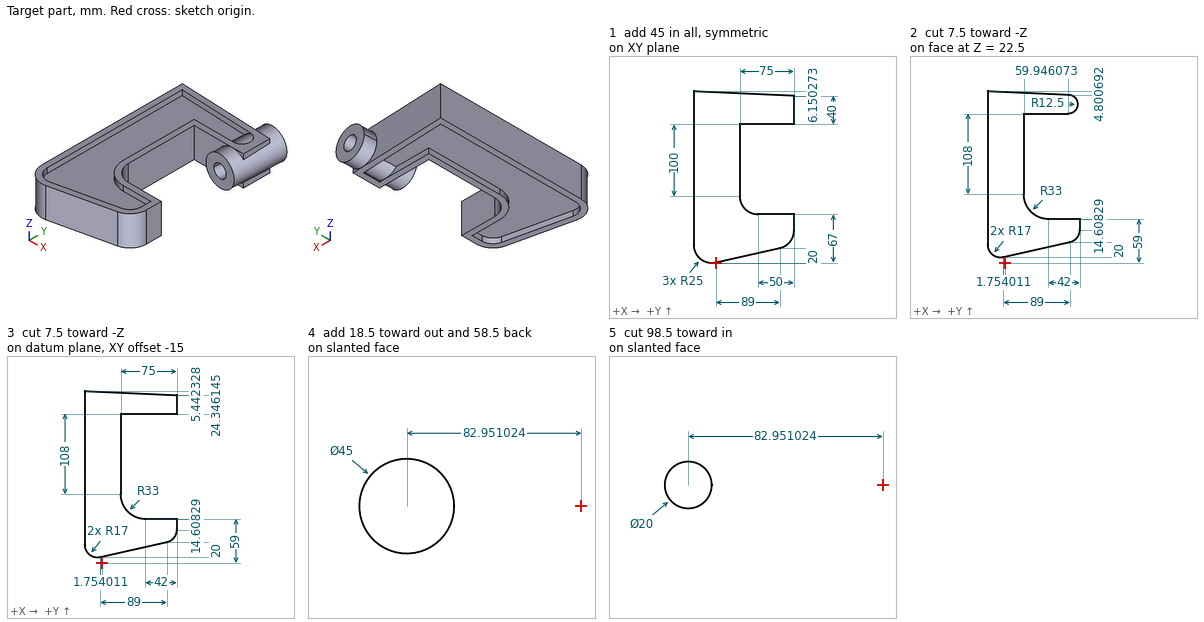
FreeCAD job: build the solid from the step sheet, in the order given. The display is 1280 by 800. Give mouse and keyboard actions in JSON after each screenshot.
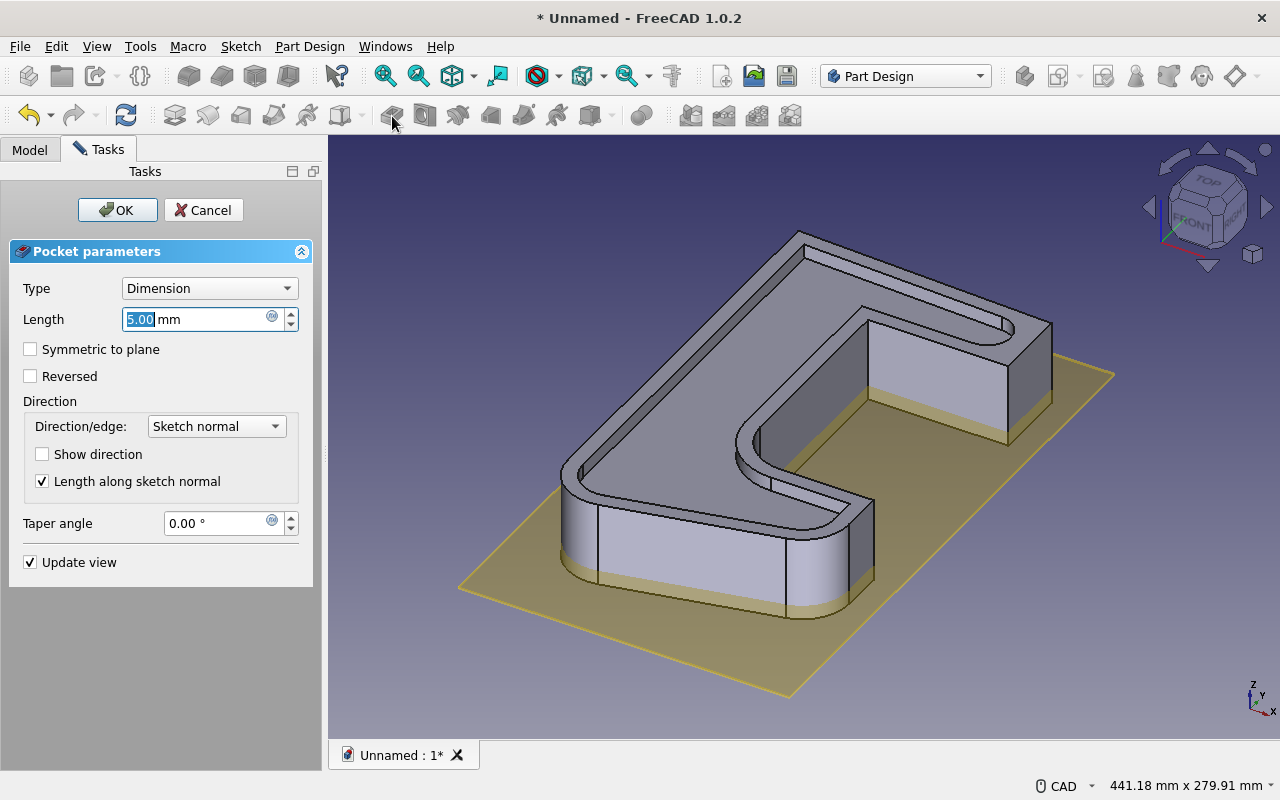
{"action": "type", "text": "7.5"}
{"action": "key", "text": "Tab"}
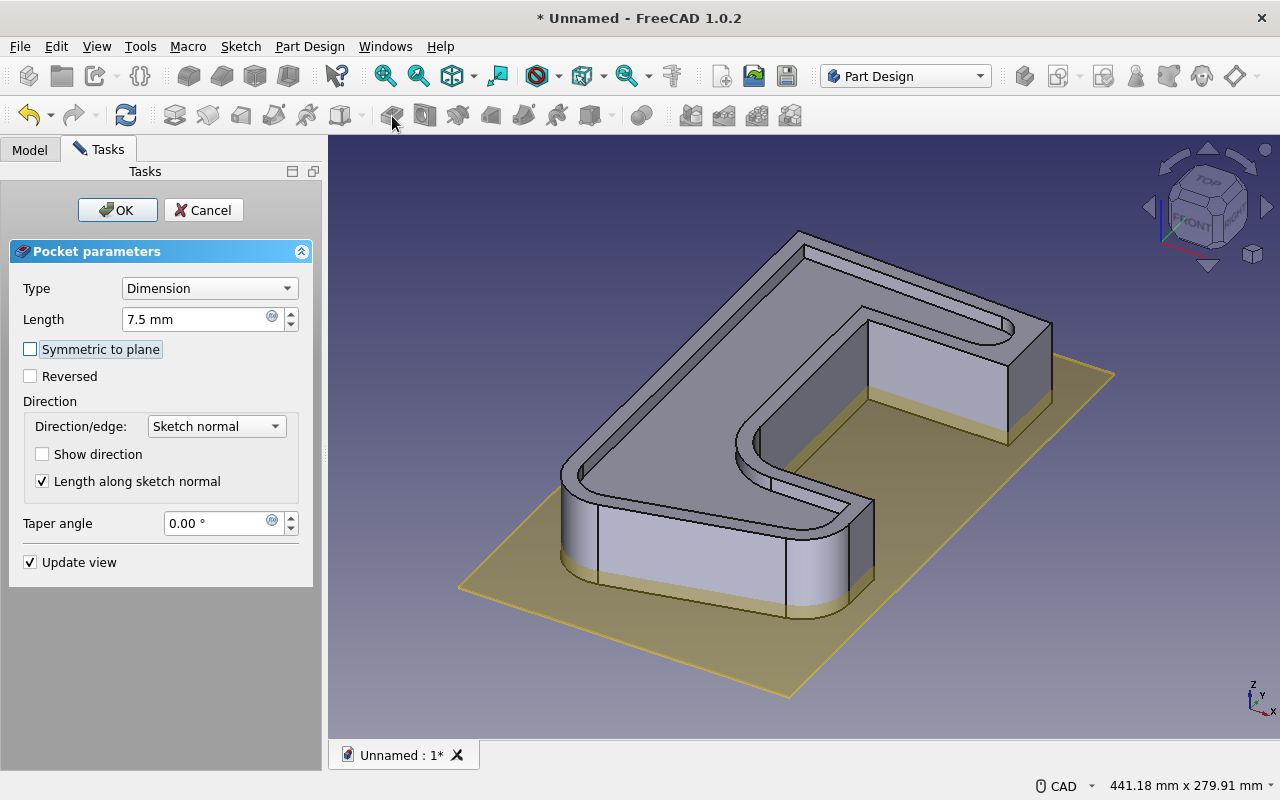
{"action": "left_click", "coordinate": [118, 210]}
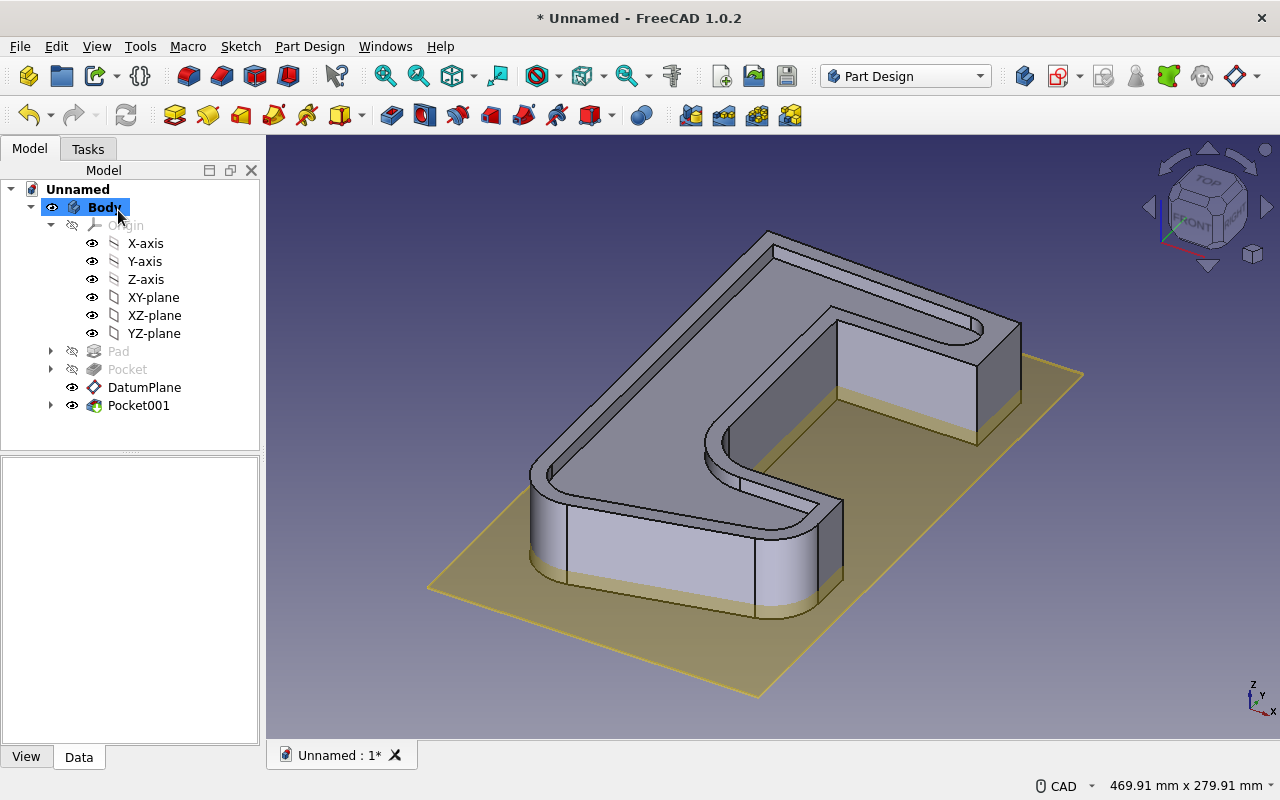
{"action": "left_click", "coordinate": [117, 387]}
{"action": "key", "text": "space"}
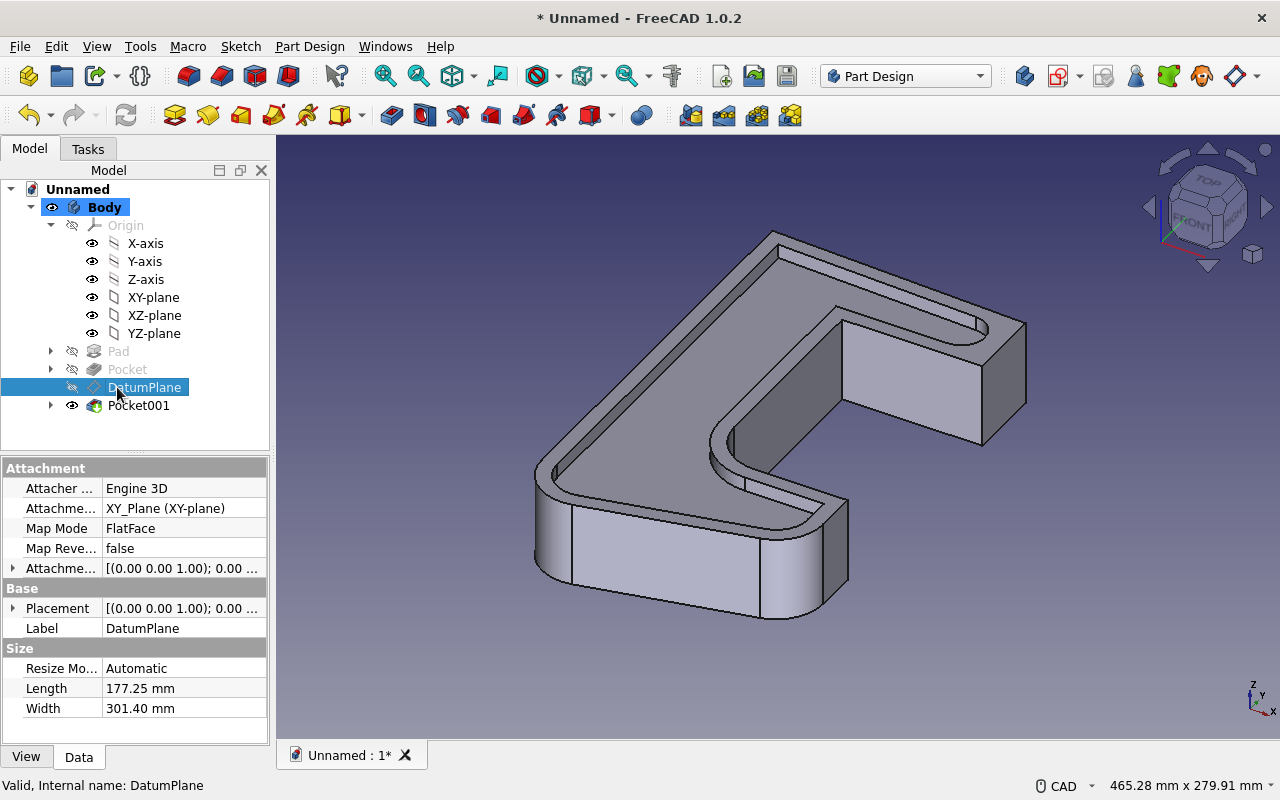
{"action": "key", "text": "4"}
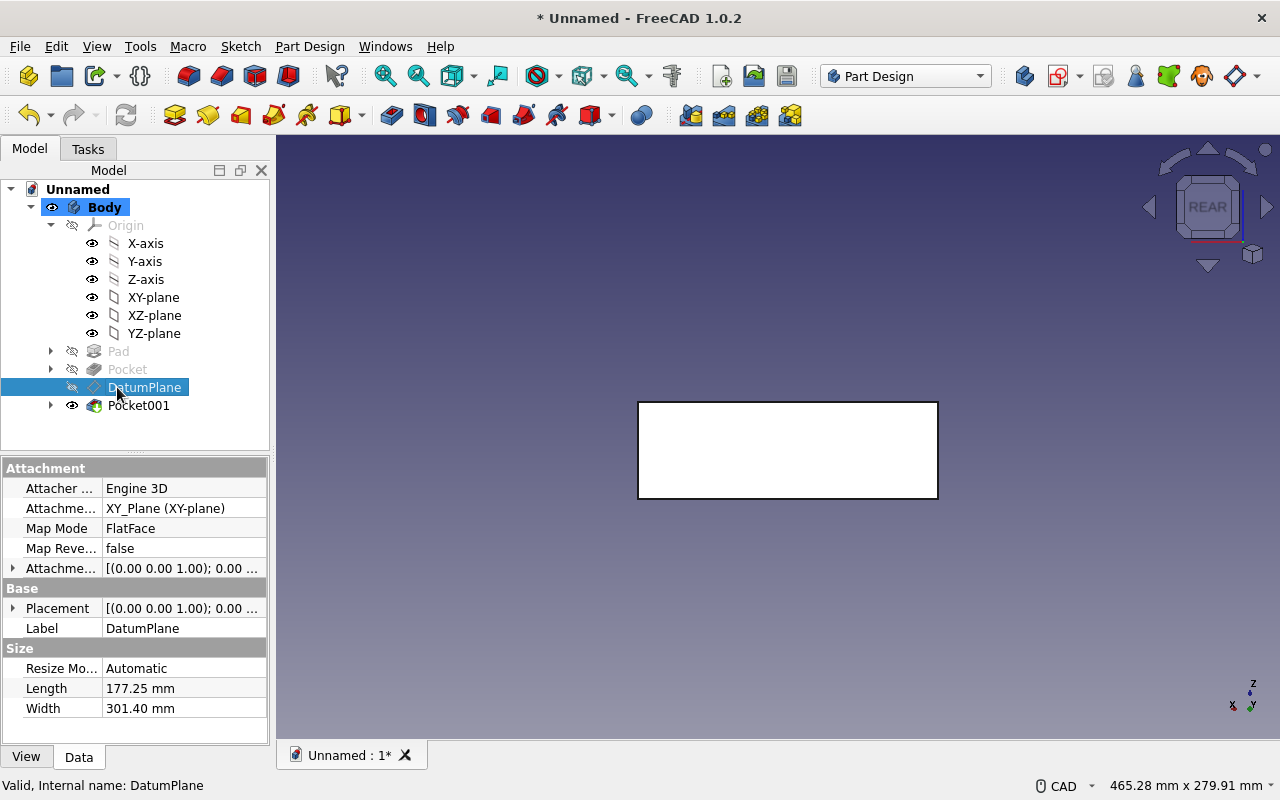
{"action": "left_click", "coordinate": [386, 76]}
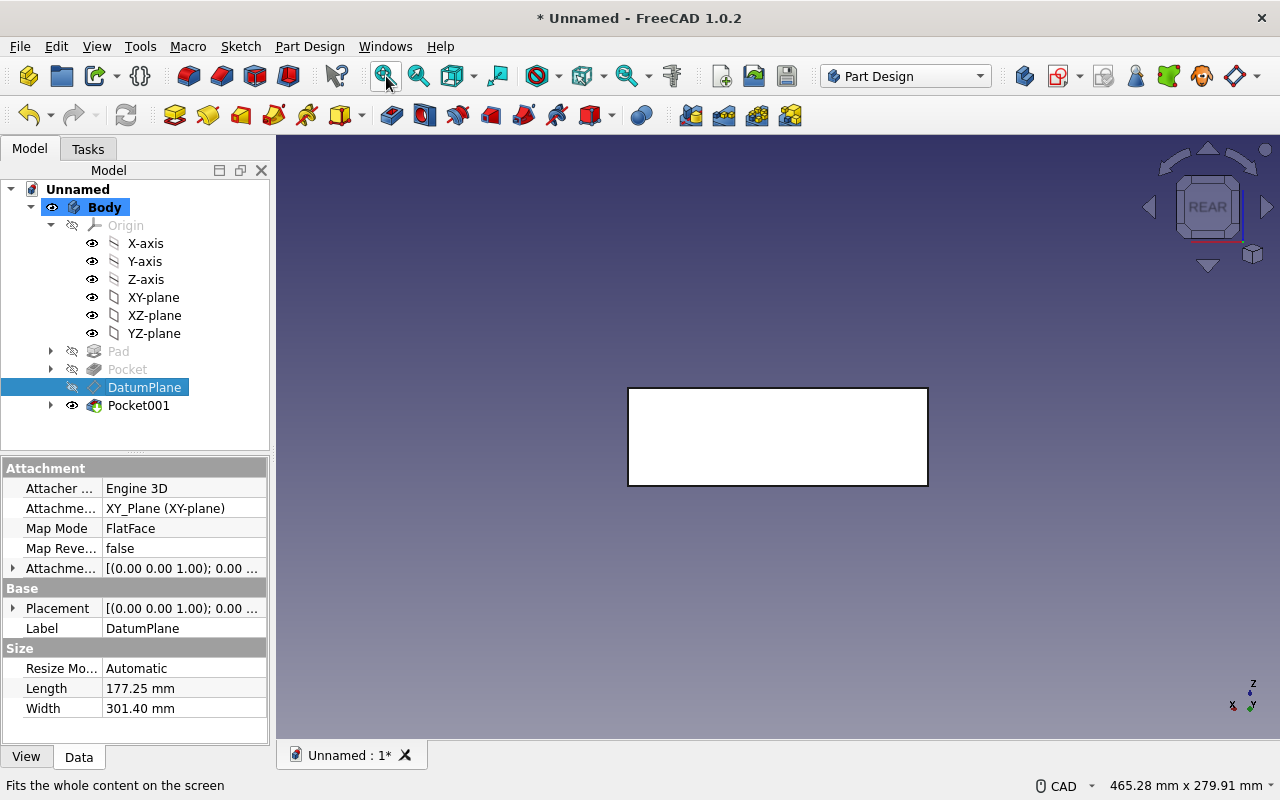
{"action": "left_click", "coordinate": [692, 436]}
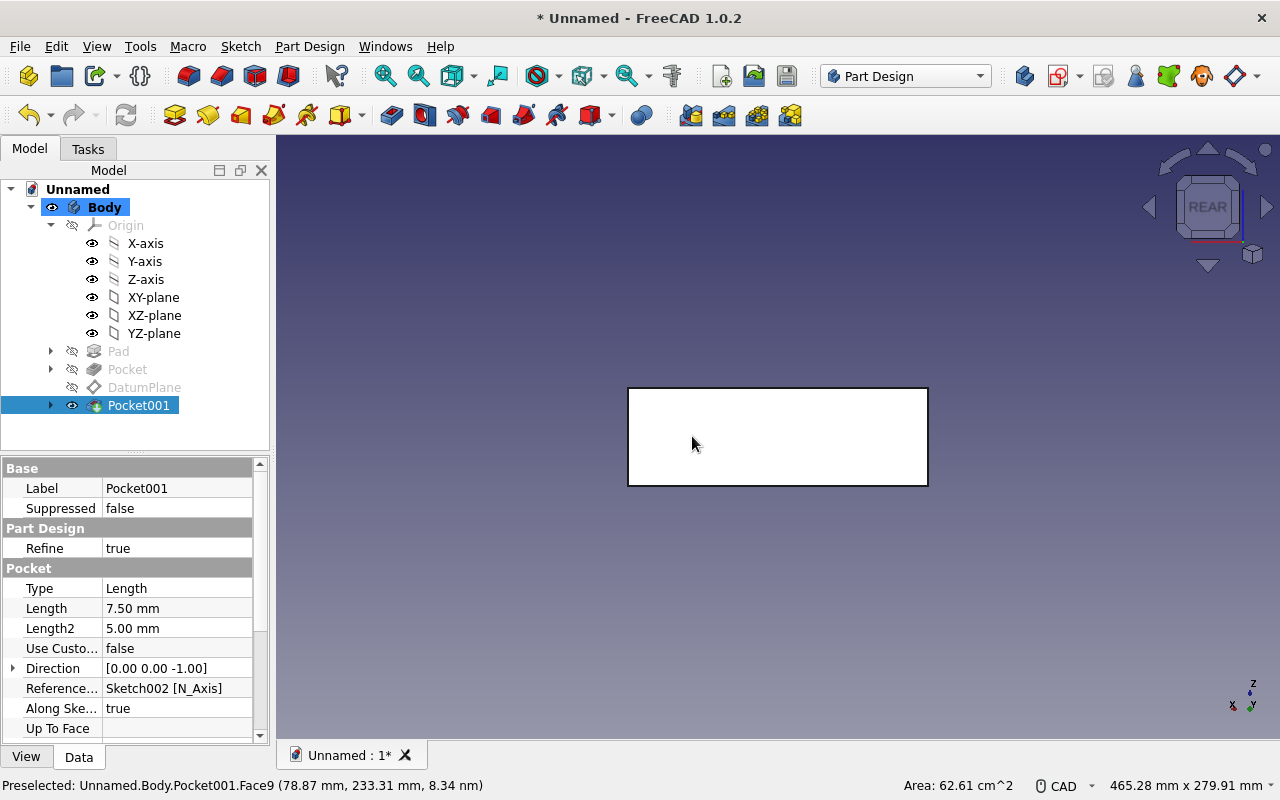
{"action": "left_click", "coordinate": [1058, 76]}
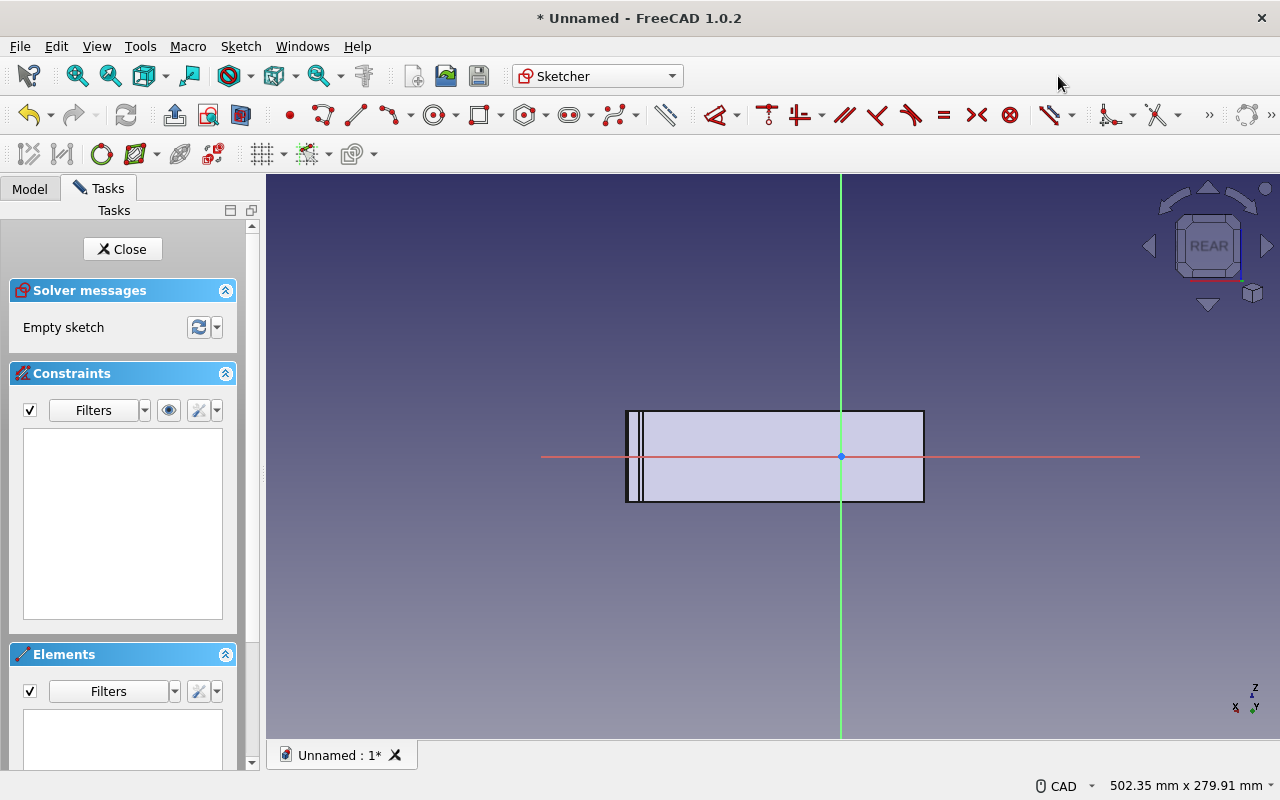
{"action": "scroll", "coordinate": [752, 456], "scroll_direction": "up", "scroll_amount": 5}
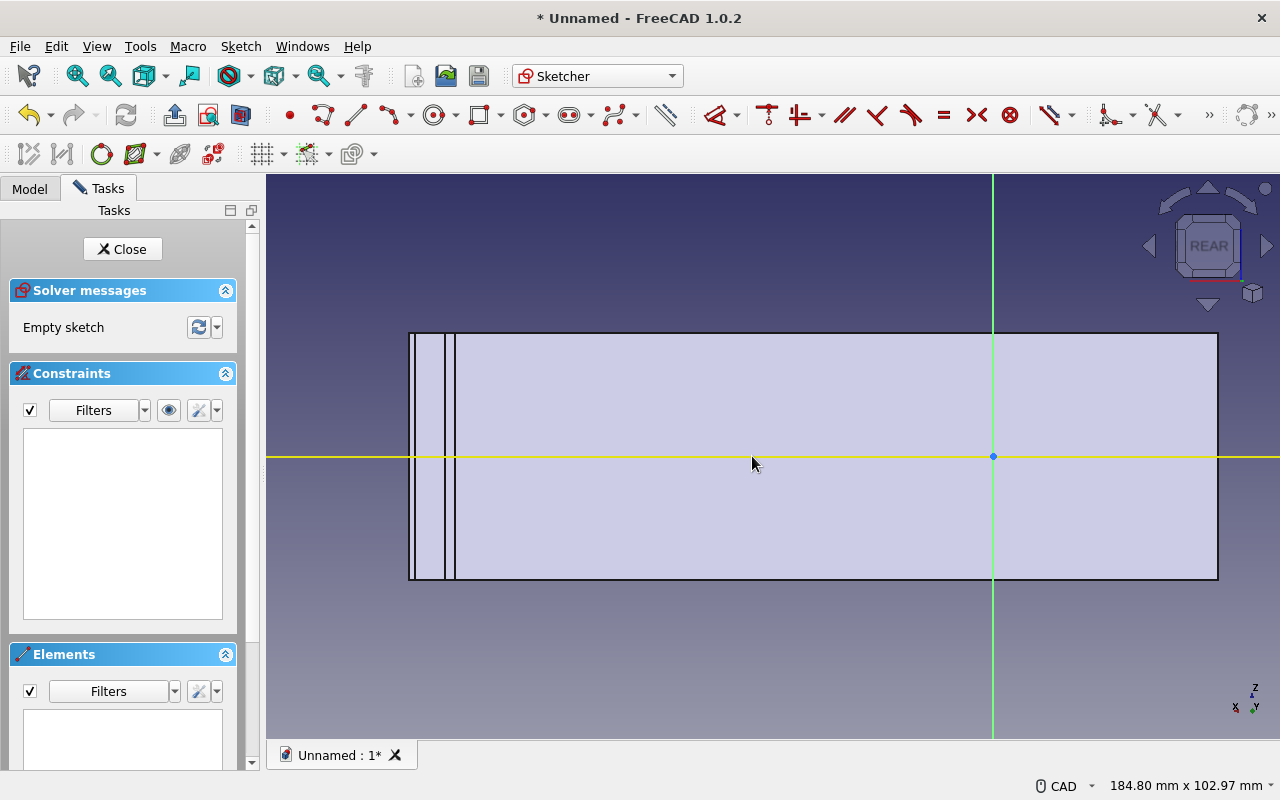
{"action": "left_click", "coordinate": [434, 116]}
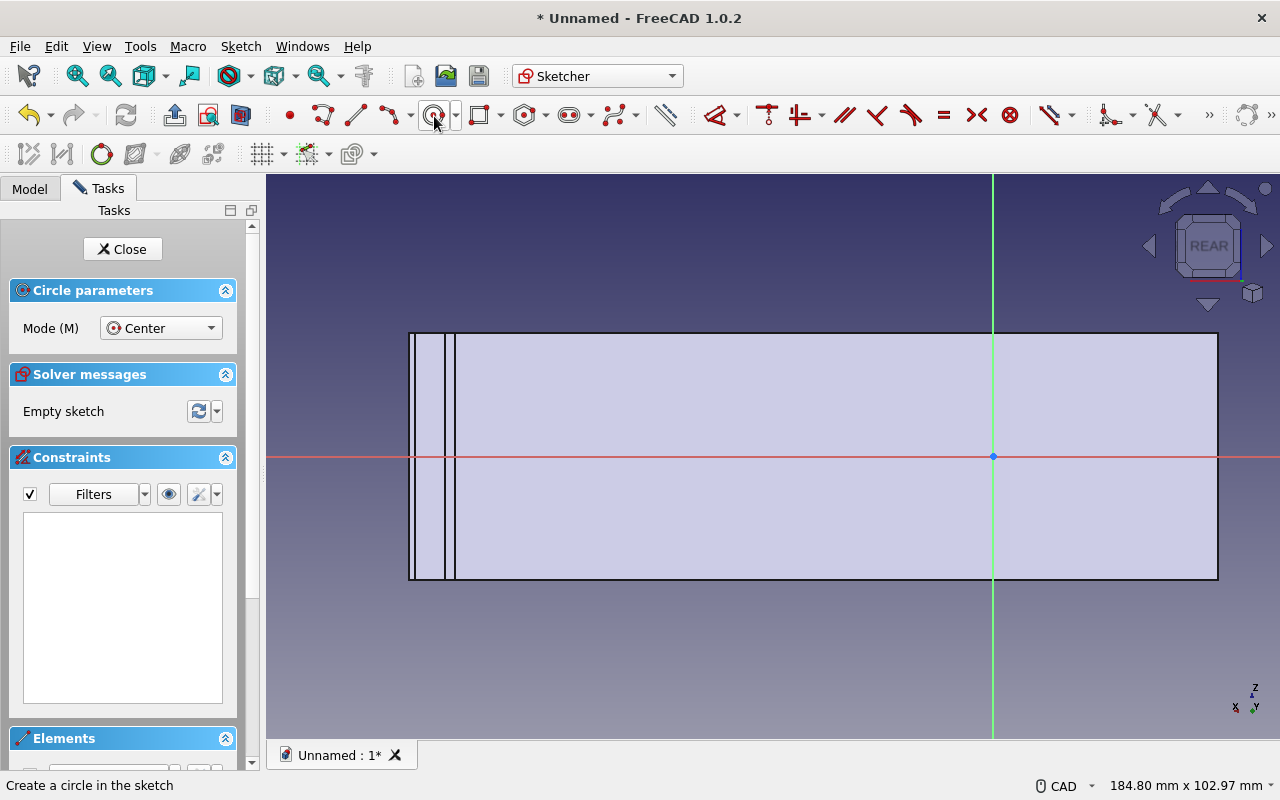
{"action": "left_click", "coordinate": [538, 456]}
{"action": "left_click", "coordinate": [625, 369]}
{"action": "key", "text": "Escape"}